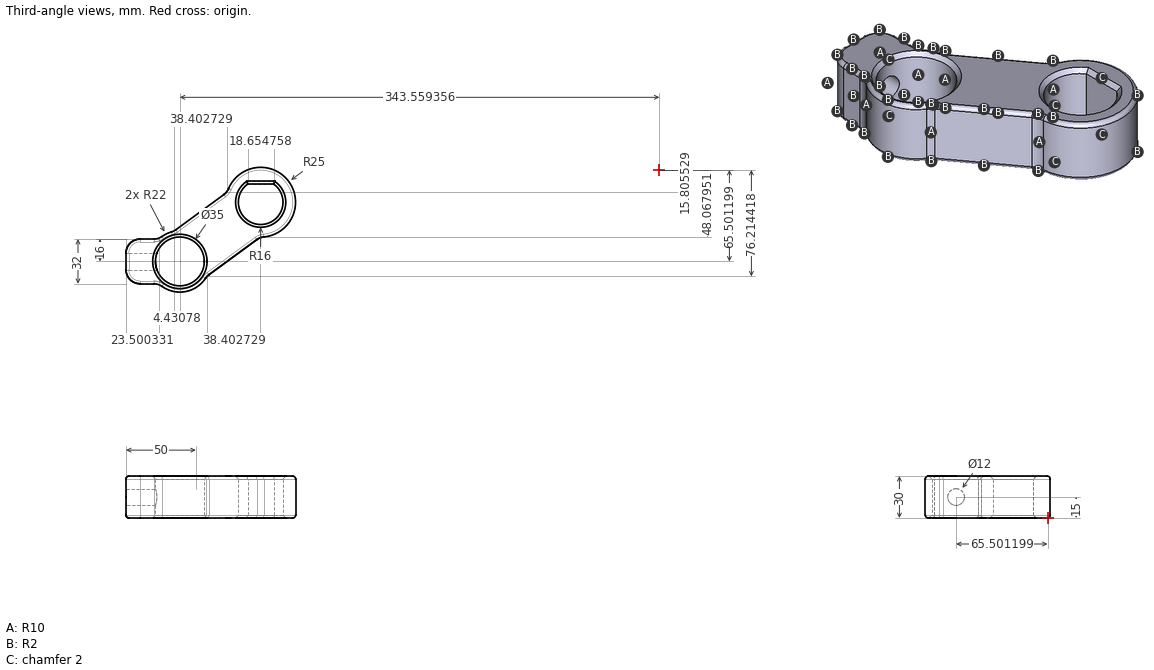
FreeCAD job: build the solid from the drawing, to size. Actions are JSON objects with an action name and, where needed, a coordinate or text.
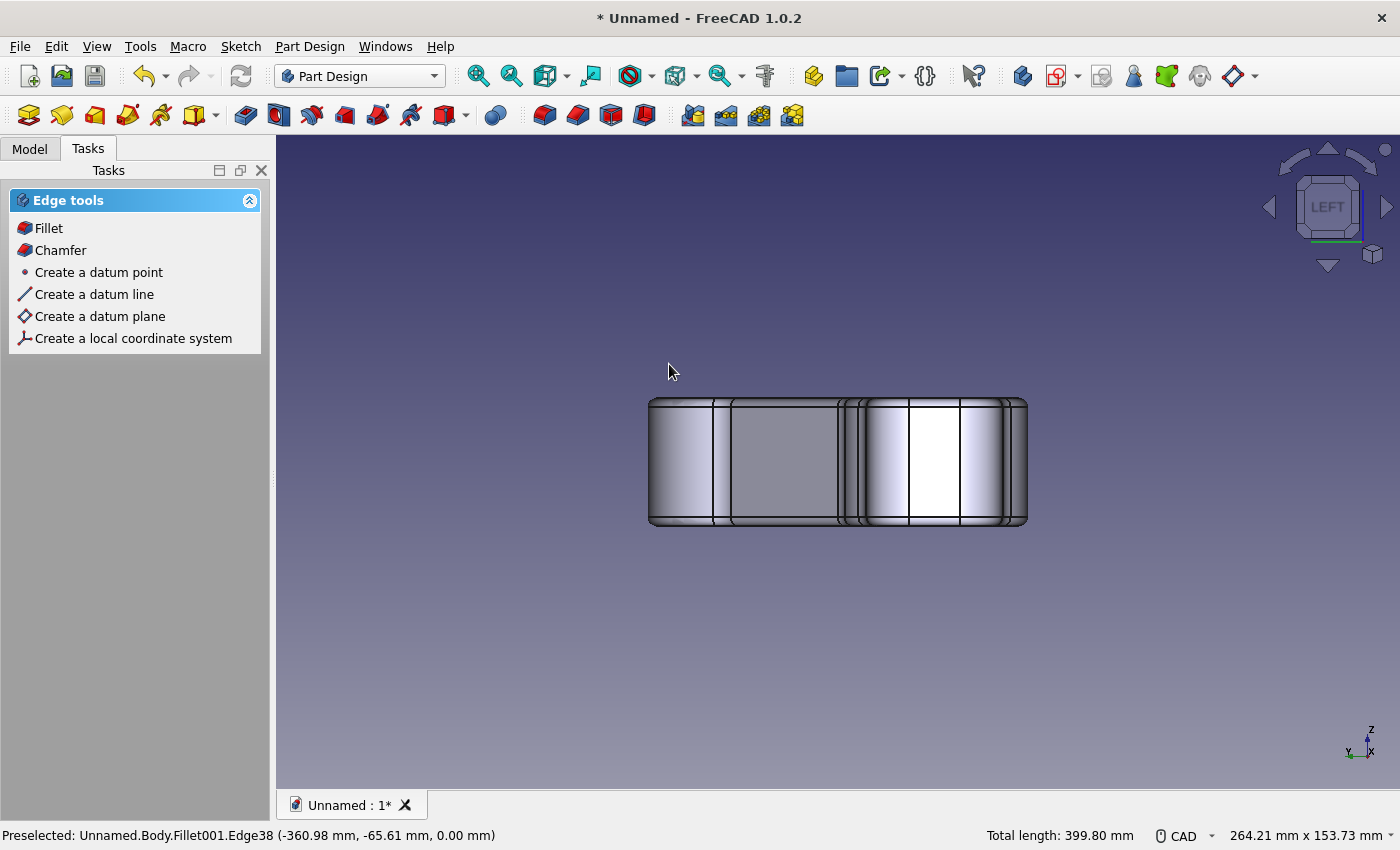
{"action": "left_click", "coordinate": [479, 76]}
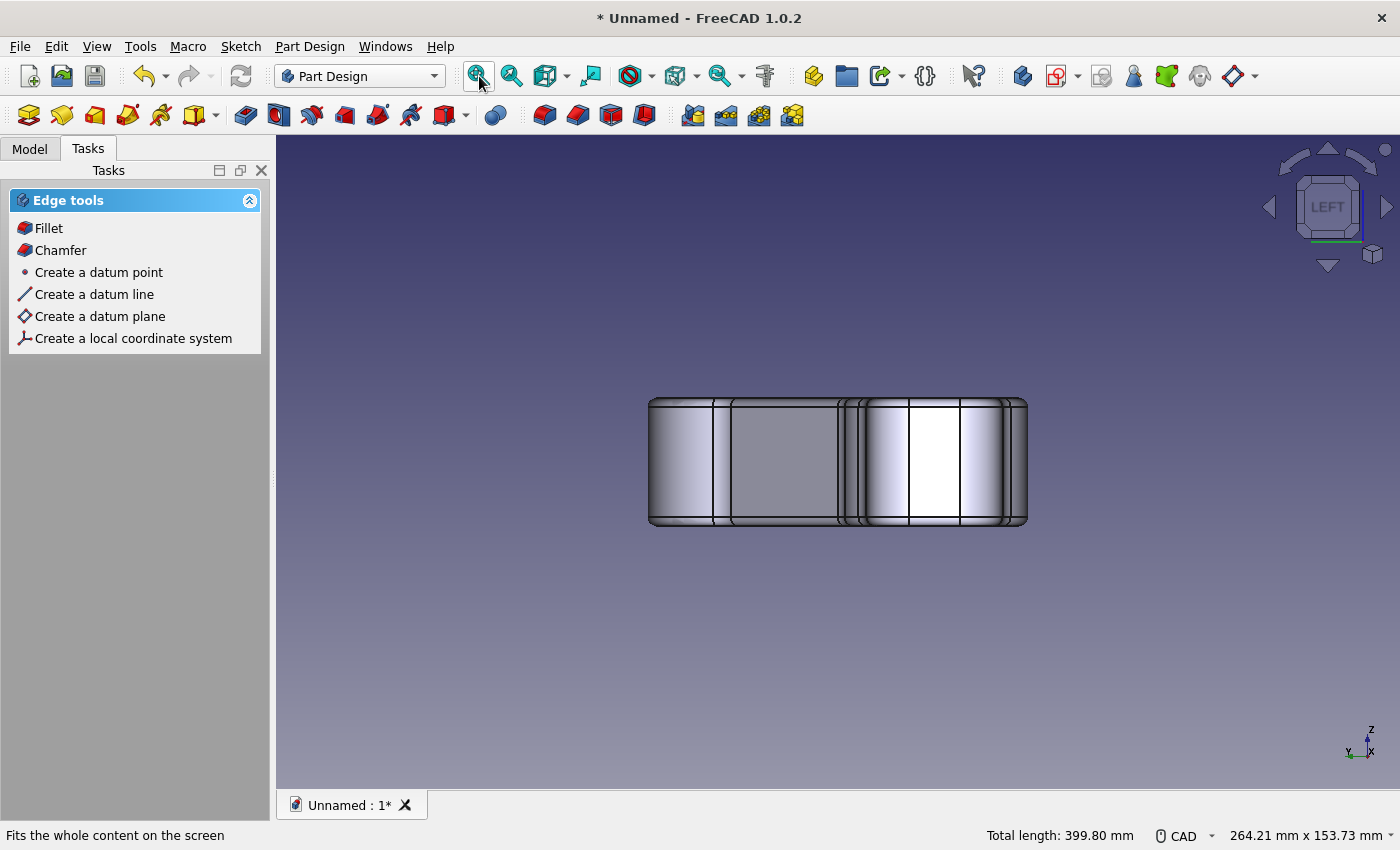
{"action": "key", "text": "v 3"}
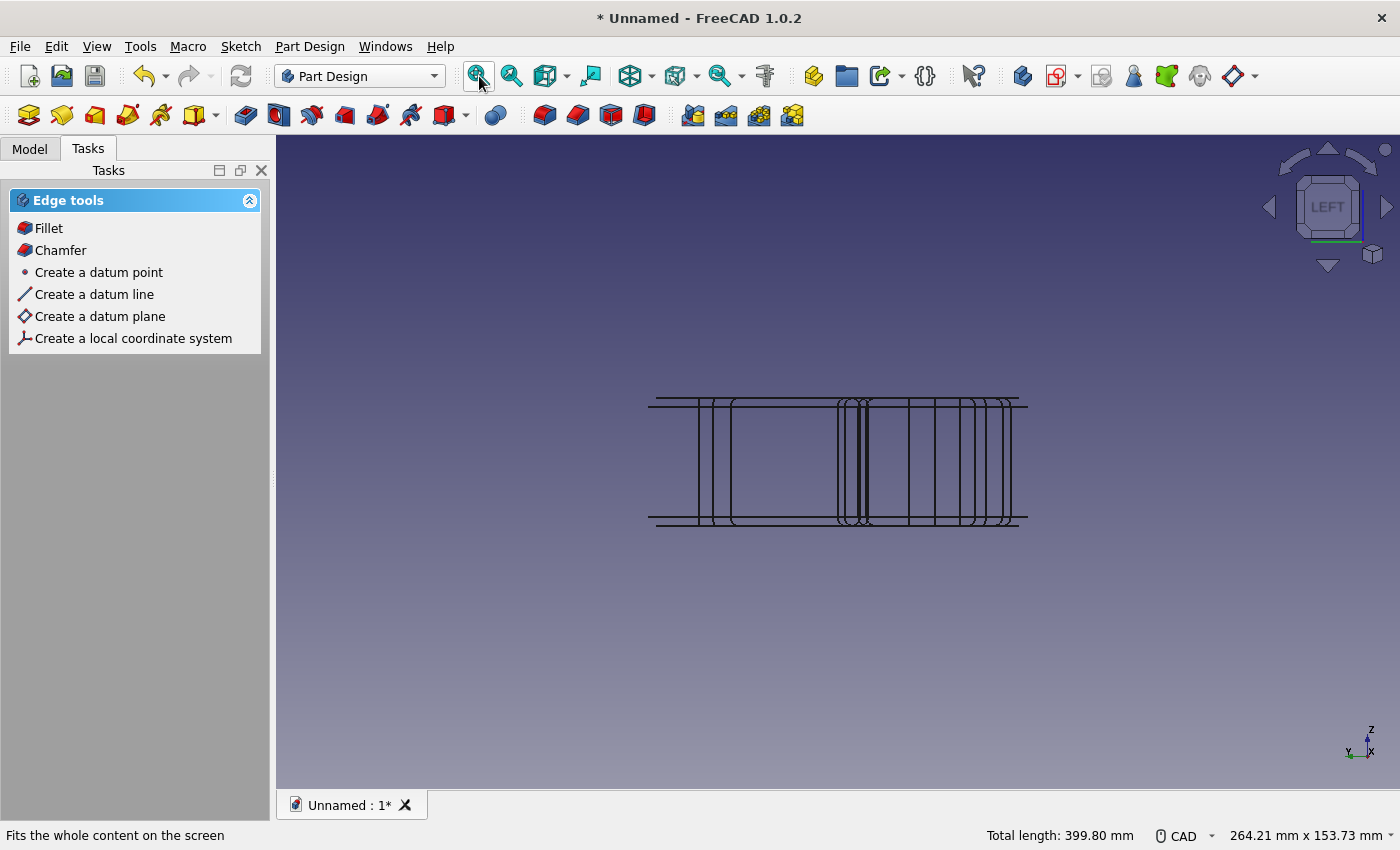
{"action": "key", "text": "0"}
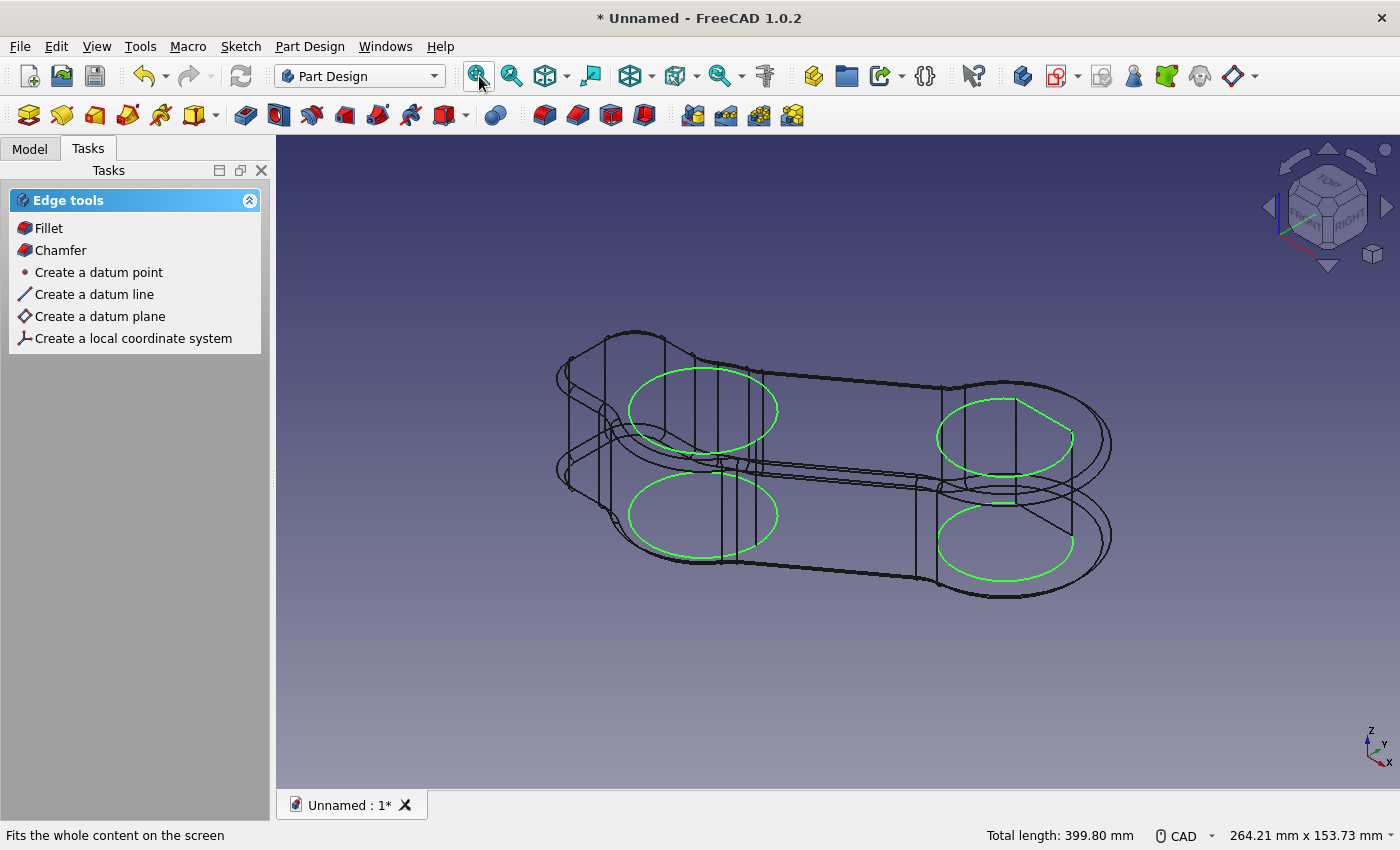
{"action": "left_click", "coordinate": [1044, 518], "text": "ctrl"}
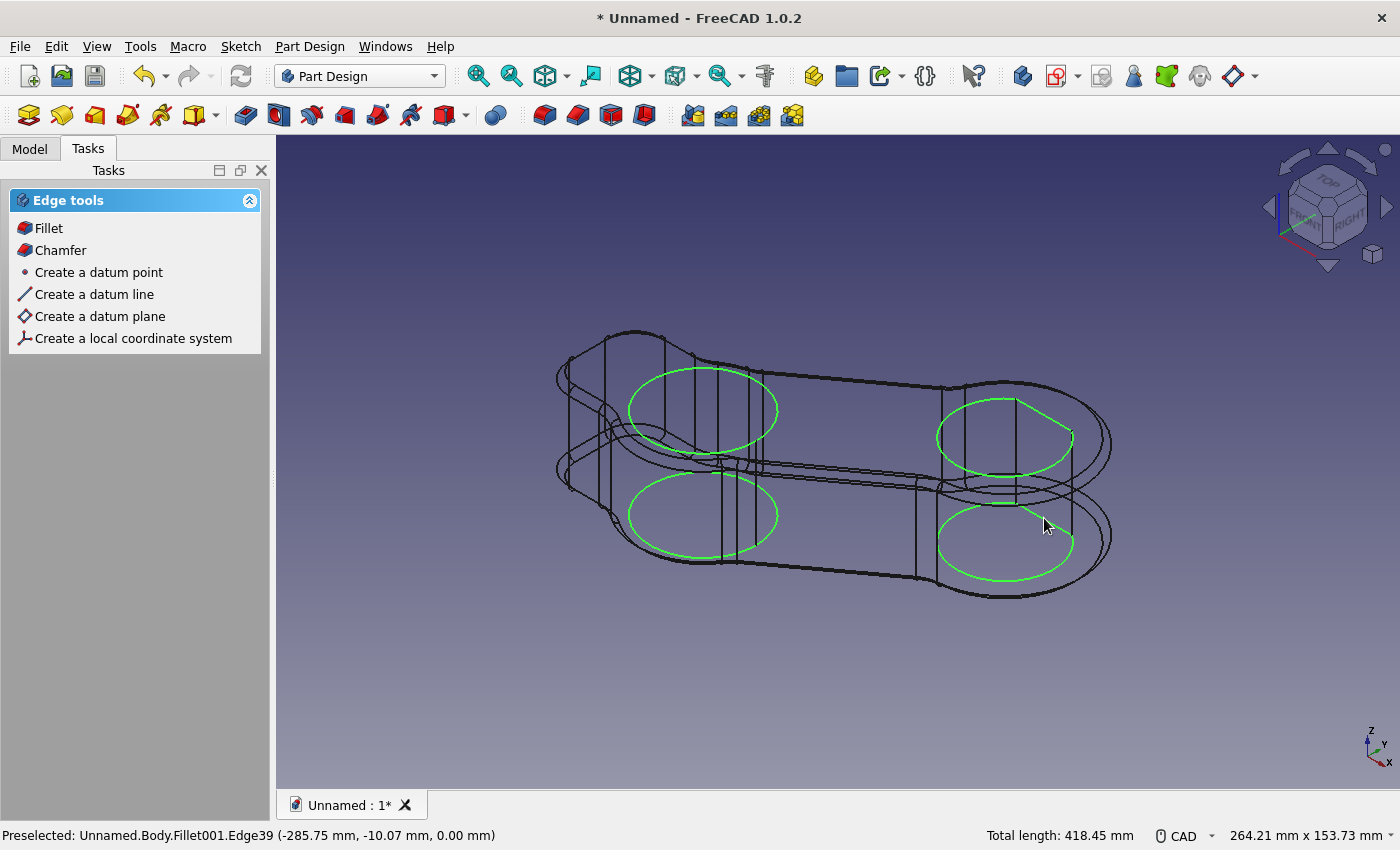
{"action": "key", "text": "v 1"}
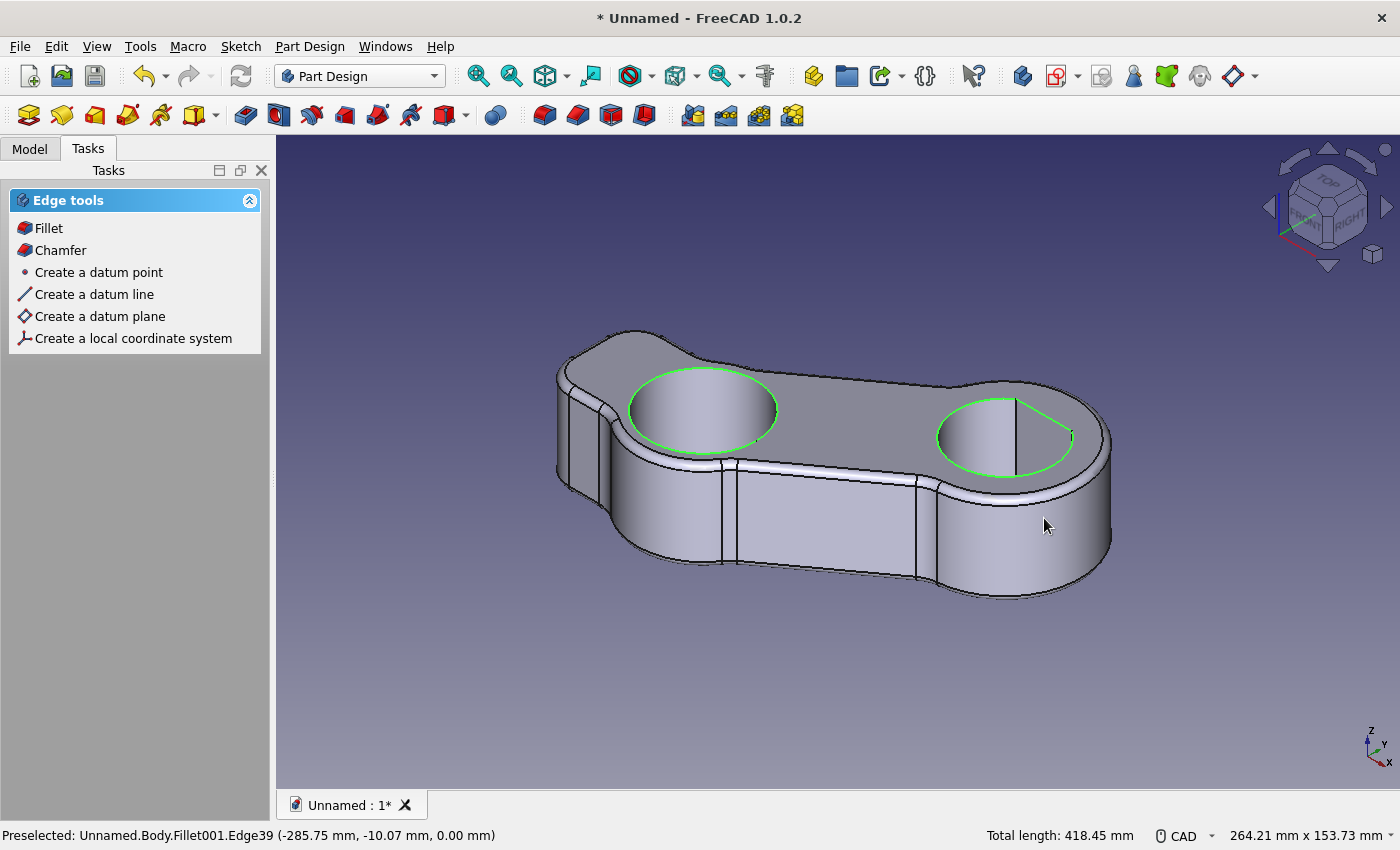
{"action": "left_click", "coordinate": [578, 116]}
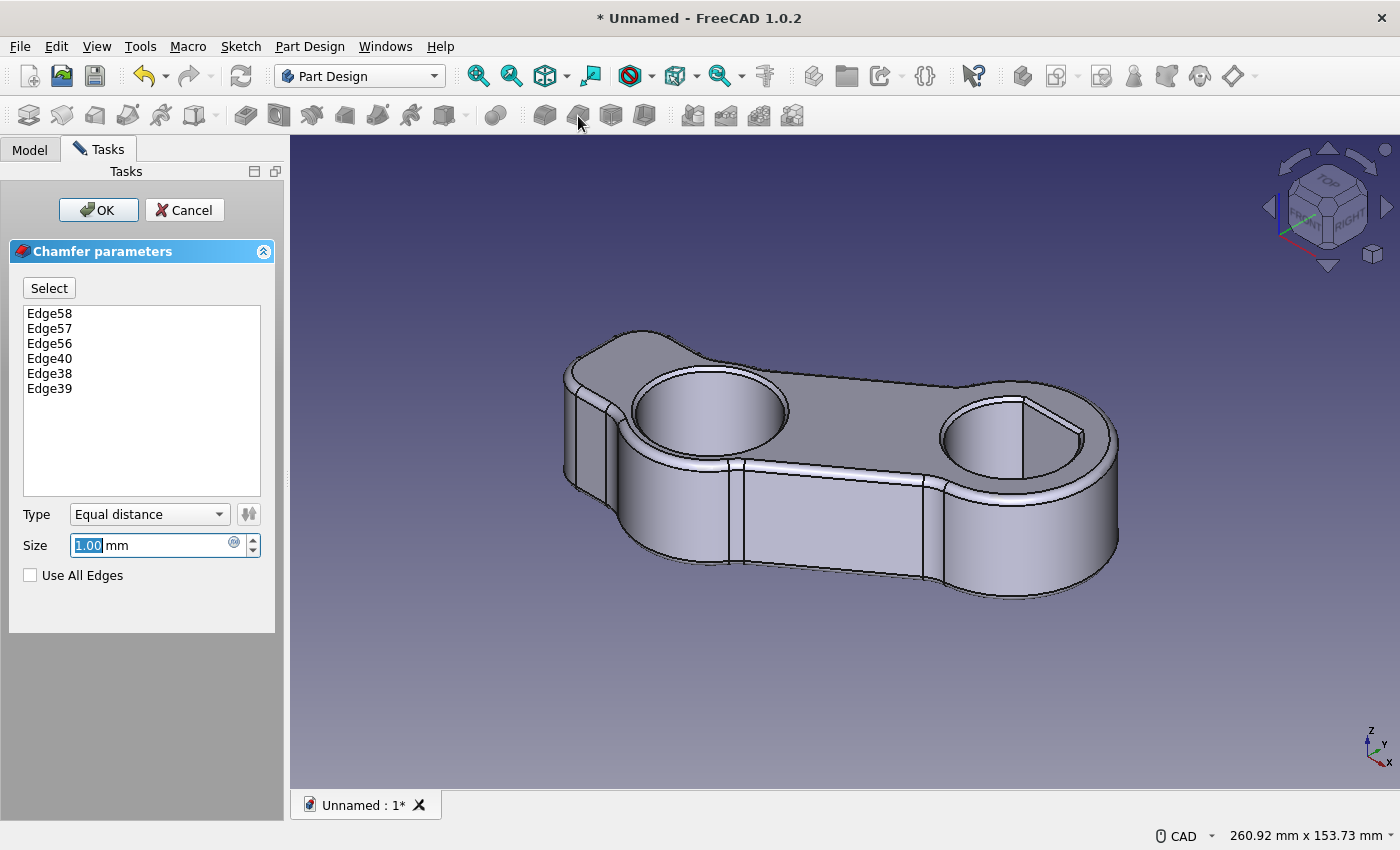
{"action": "type", "text": "2"}
{"action": "key", "text": "Tab"}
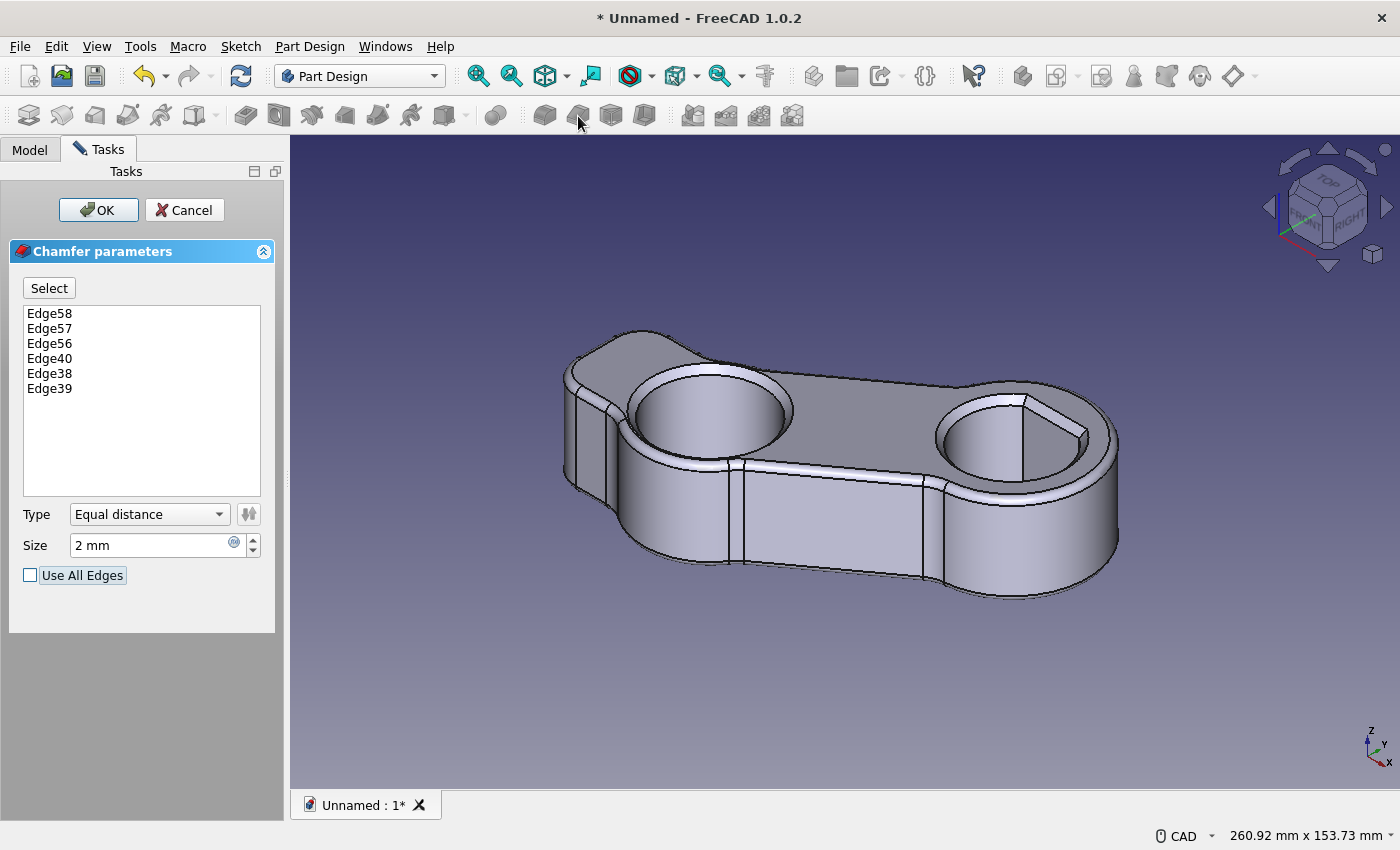
{"action": "left_click", "coordinate": [99, 210]}